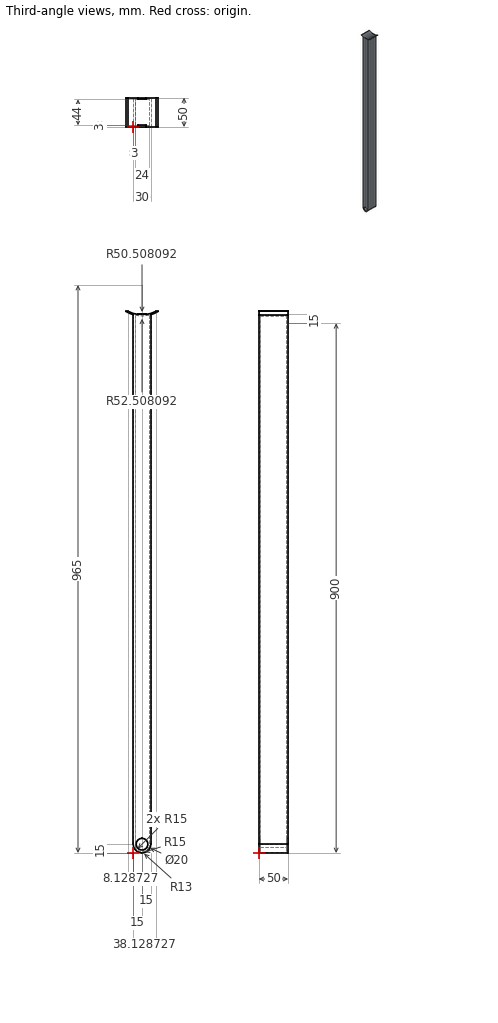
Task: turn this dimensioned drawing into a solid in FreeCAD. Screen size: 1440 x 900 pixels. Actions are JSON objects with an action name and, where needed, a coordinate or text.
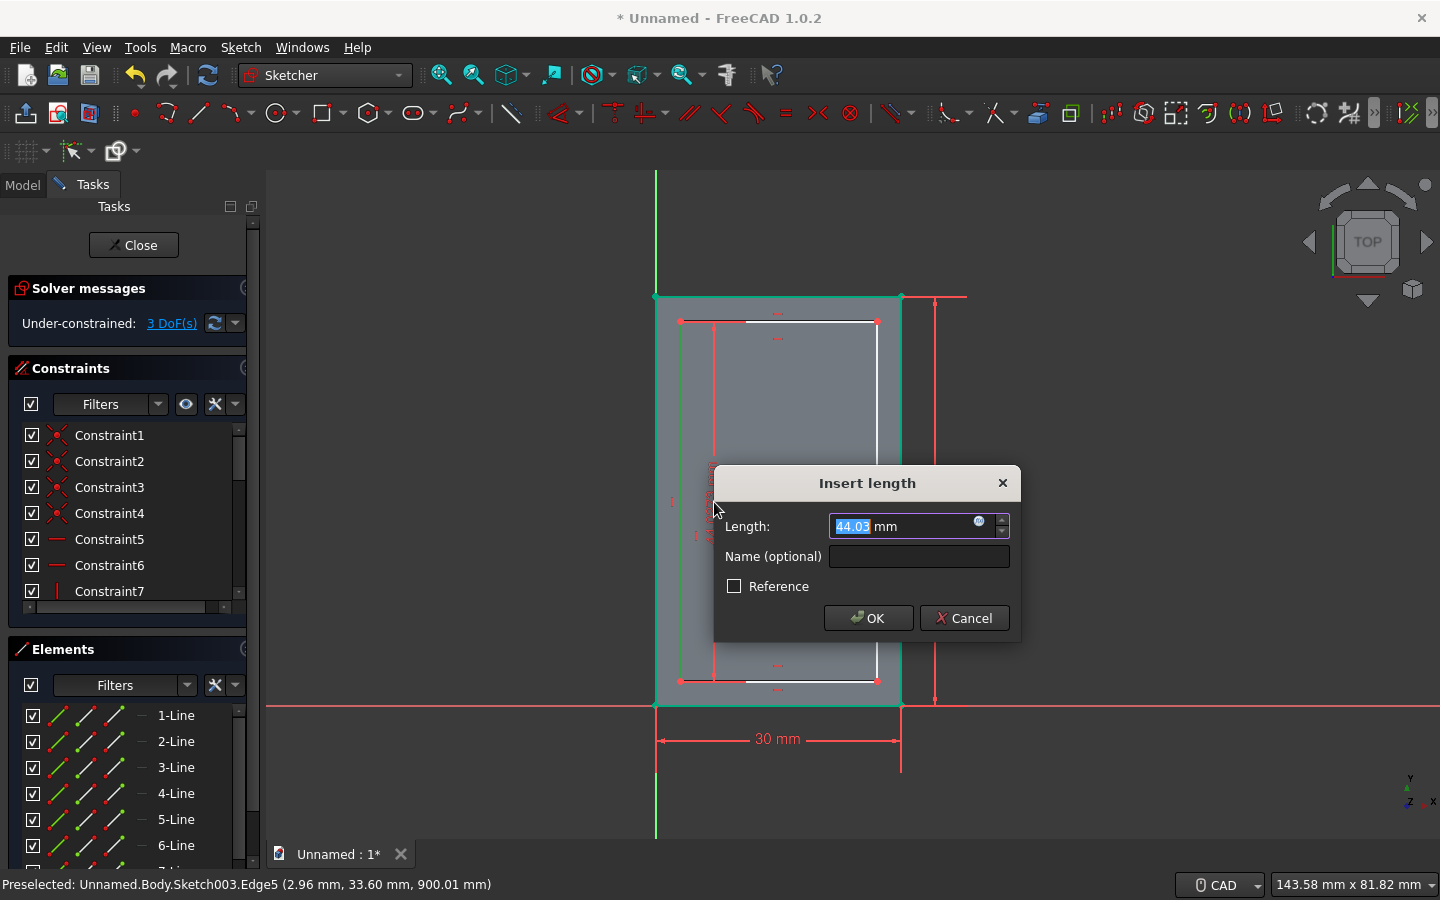
{"action": "type", "text": "44"}
{"action": "key", "text": "Return"}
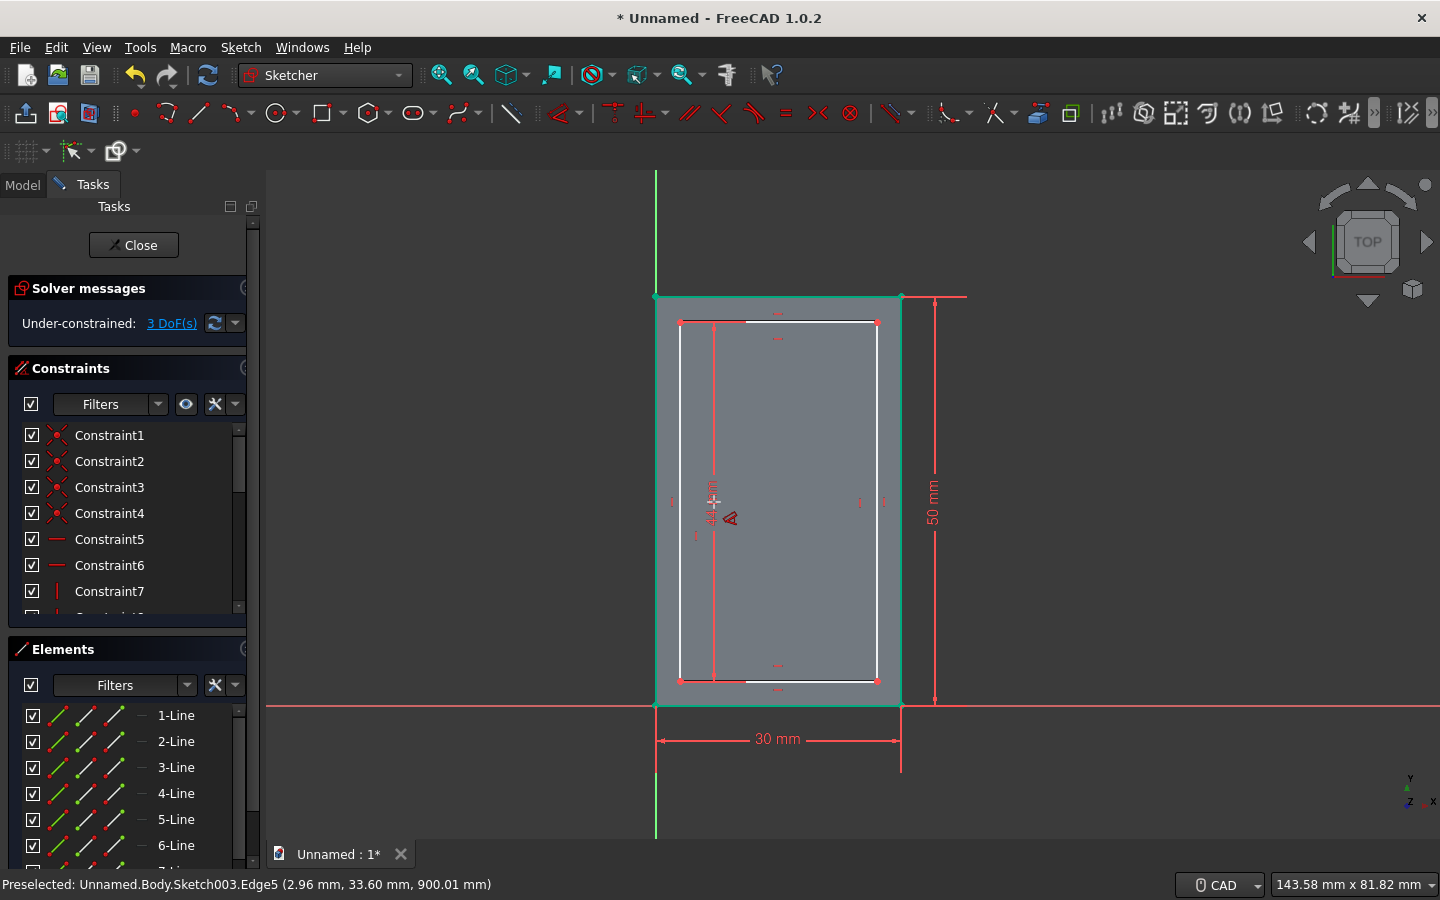
{"action": "left_click", "coordinate": [739, 682]}
{"action": "left_click", "coordinate": [778, 648]}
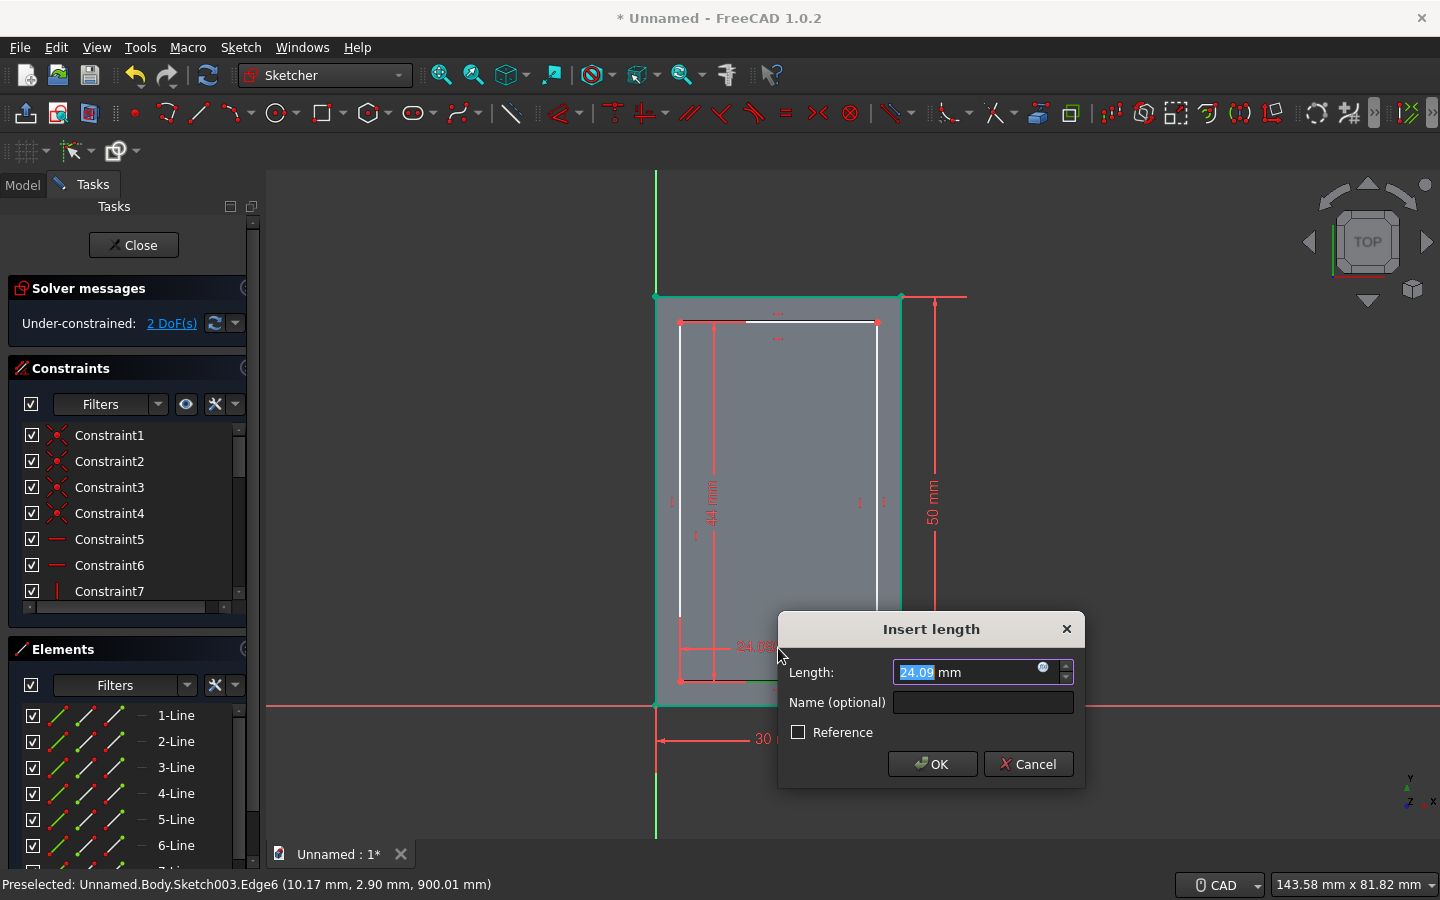
{"action": "type", "text": "24"}
{"action": "key", "text": "Return"}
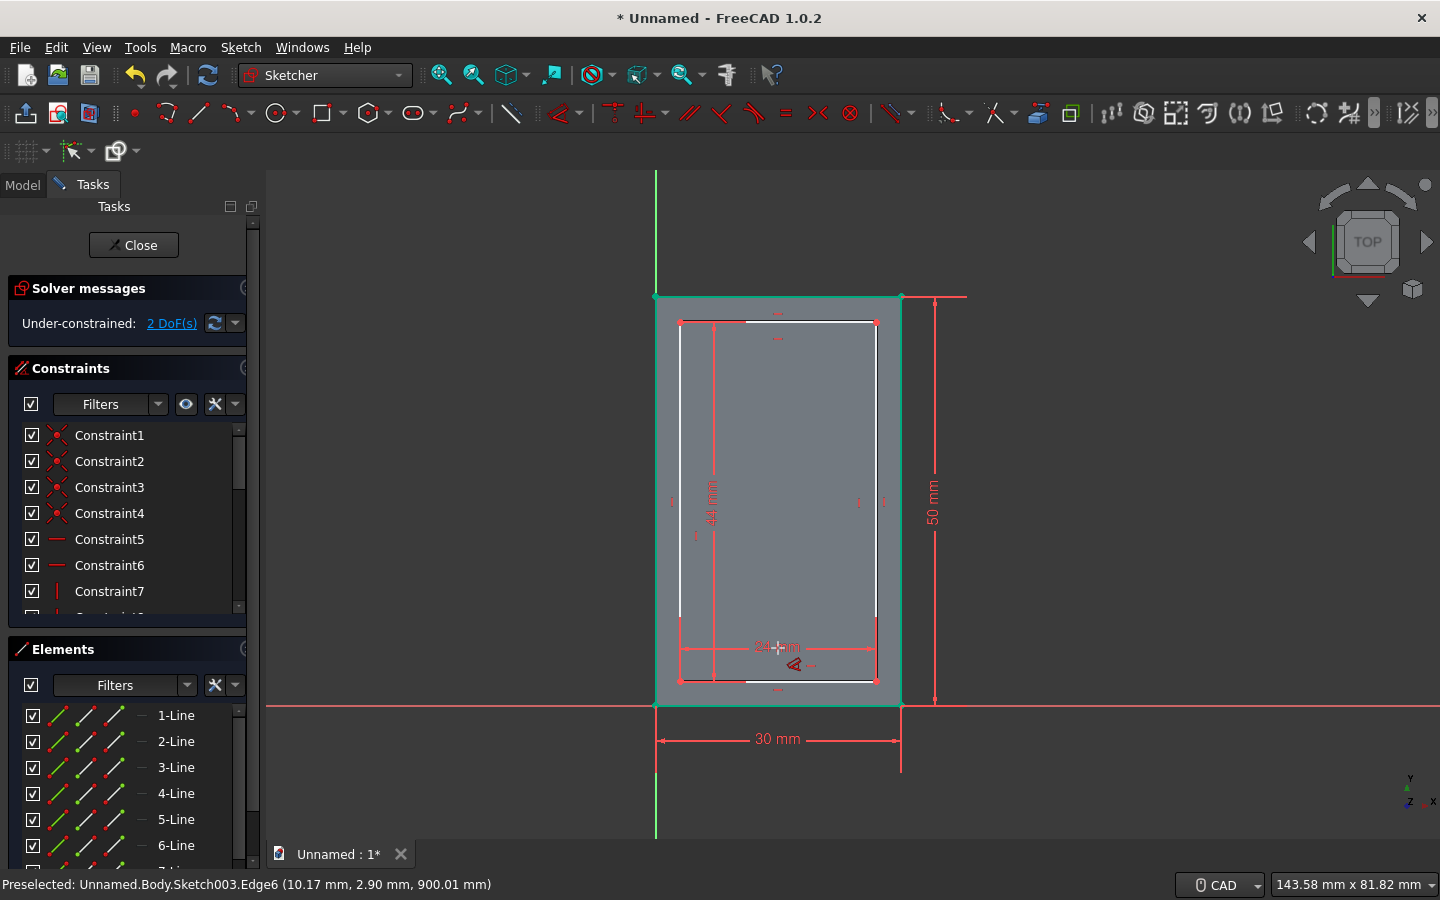
{"action": "scroll", "coordinate": [680, 322], "scroll_direction": "up", "scroll_amount": 3}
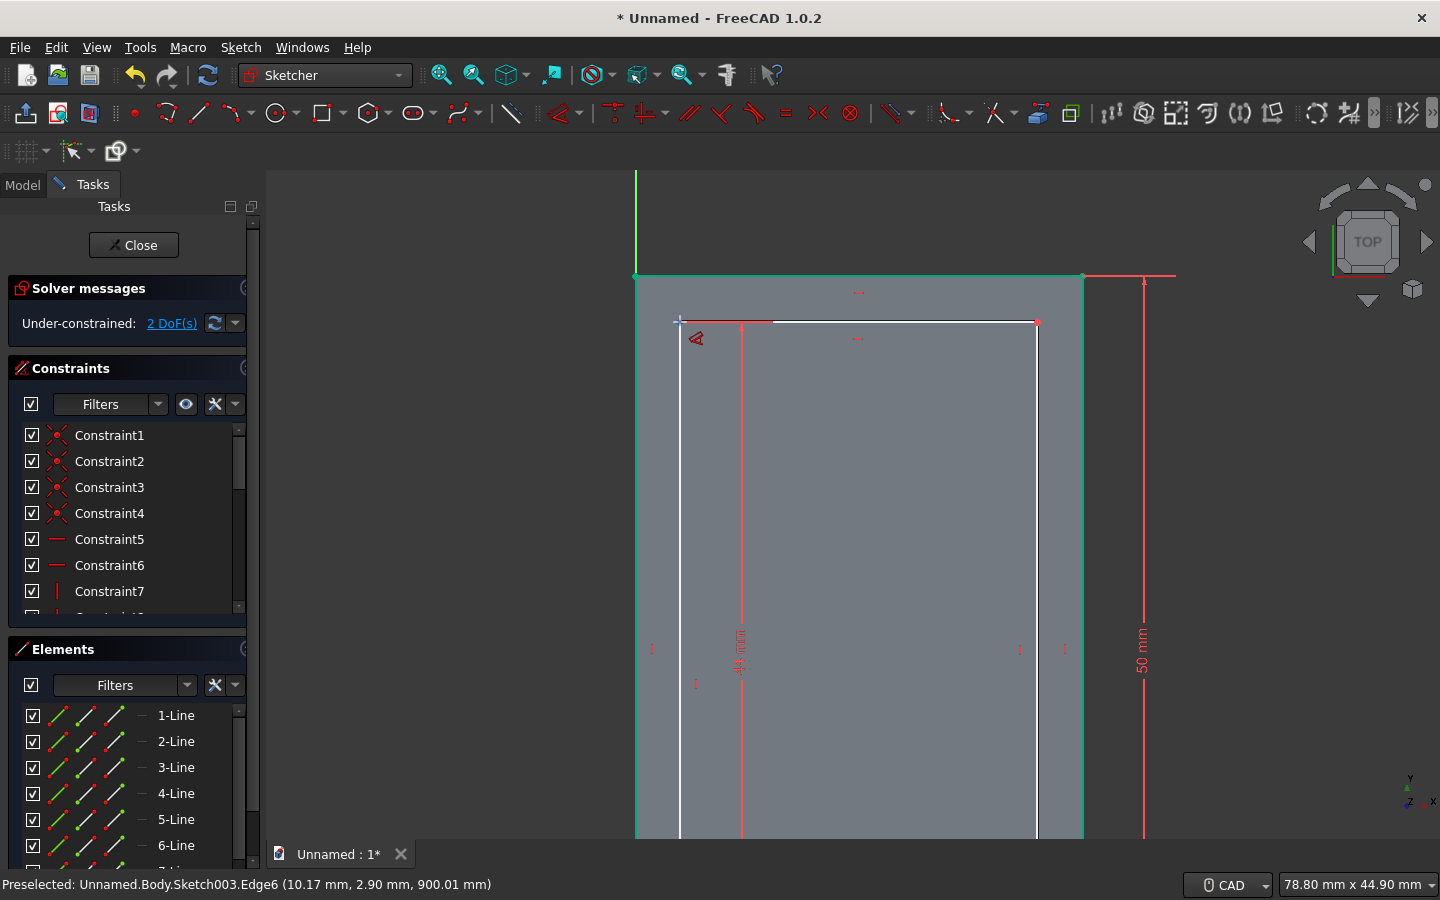
{"action": "left_click", "coordinate": [680, 322]}
{"action": "left_click", "coordinate": [658, 240]}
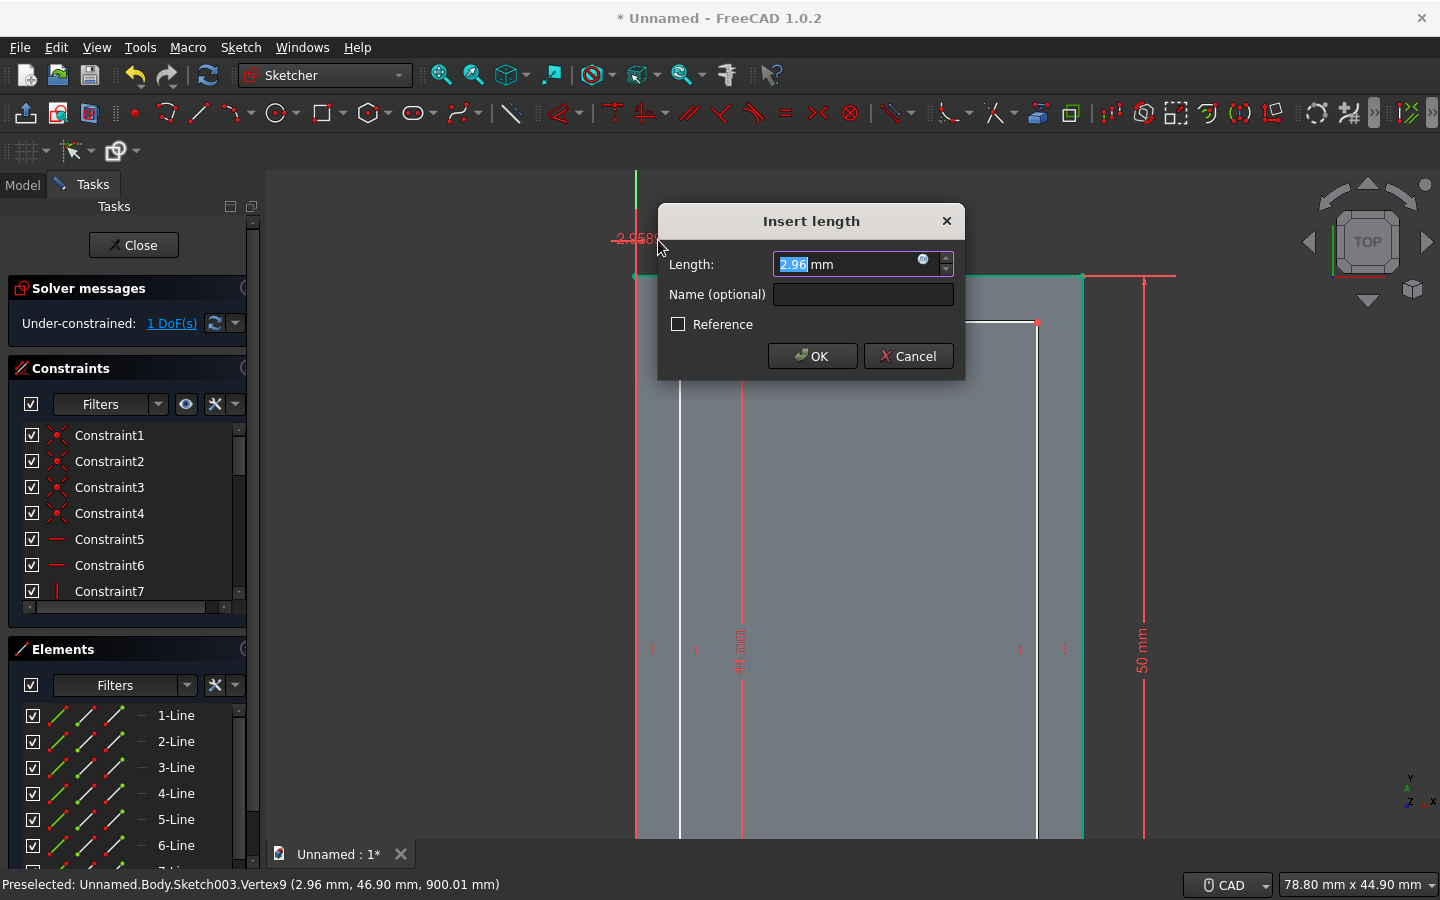
{"action": "type", "text": "3"}
{"action": "key", "text": "Return"}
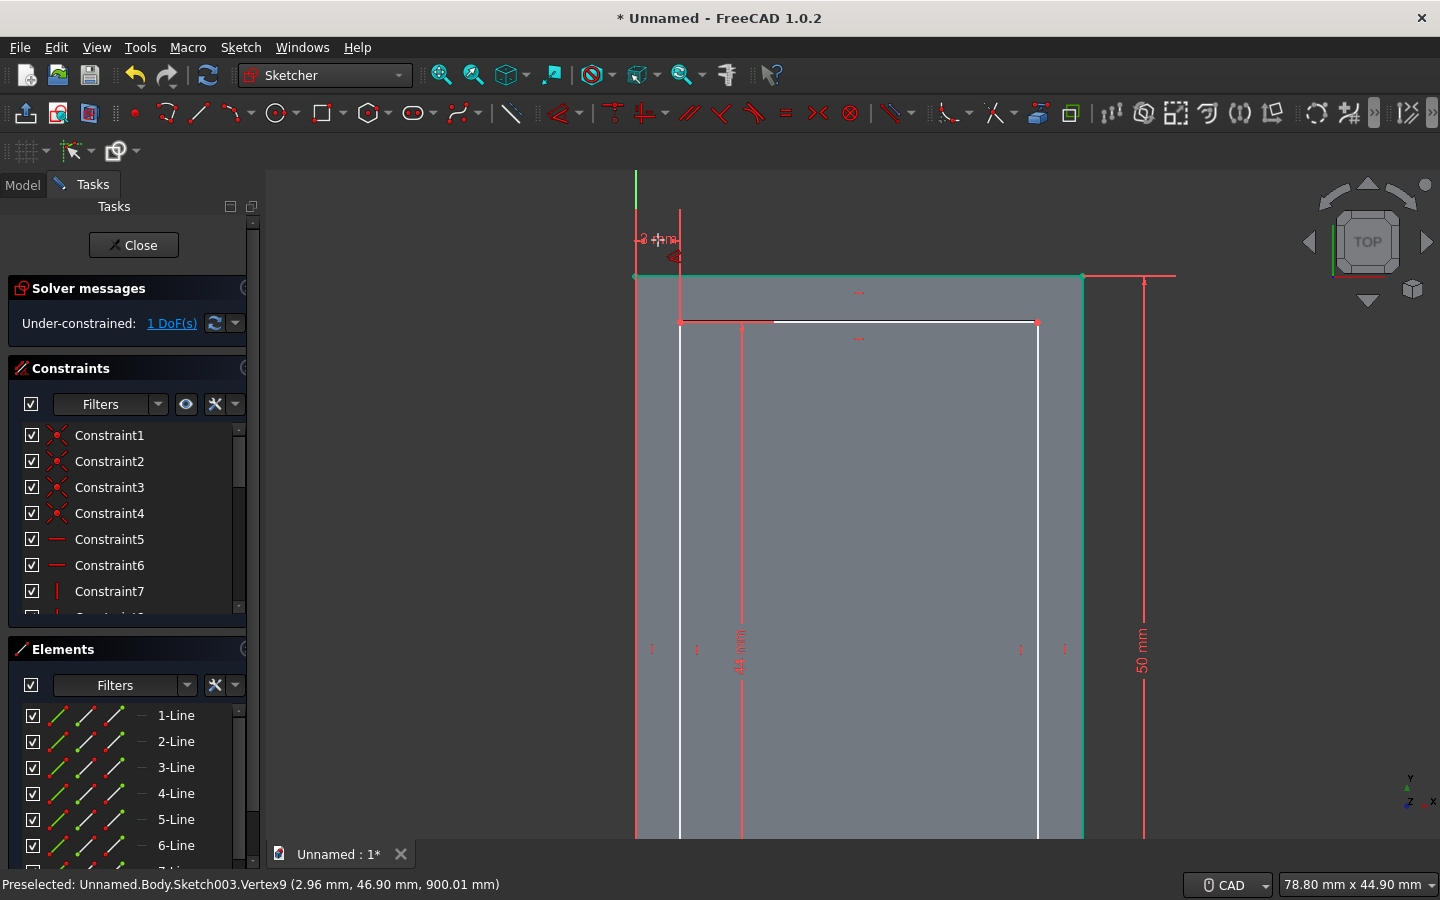
{"action": "scroll", "coordinate": [694, 329], "scroll_direction": "down", "scroll_amount": 3}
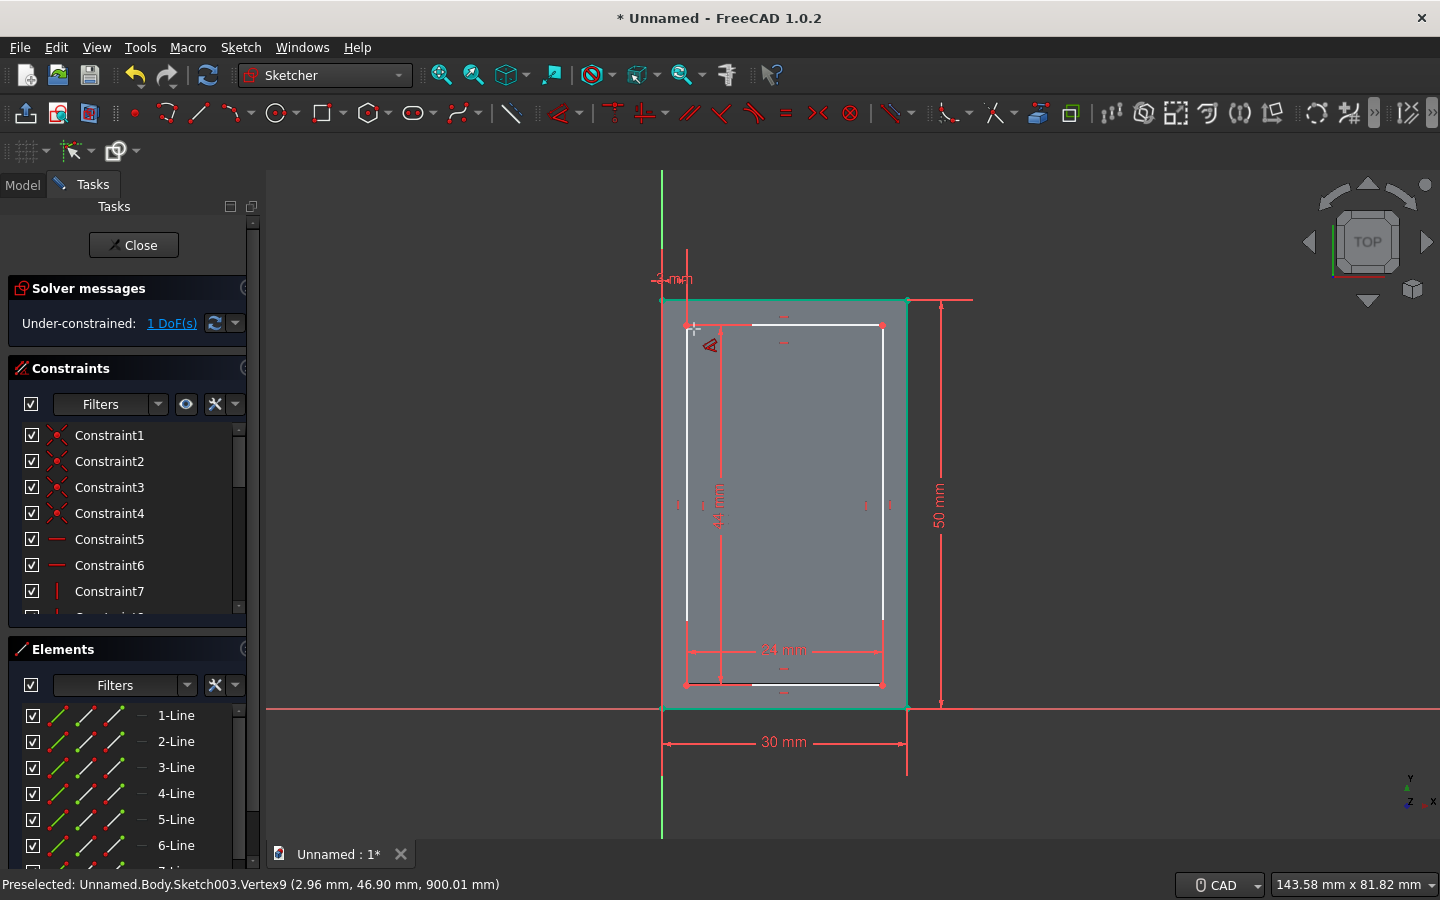
{"action": "scroll", "coordinate": [687, 685], "scroll_direction": "up", "scroll_amount": 3}